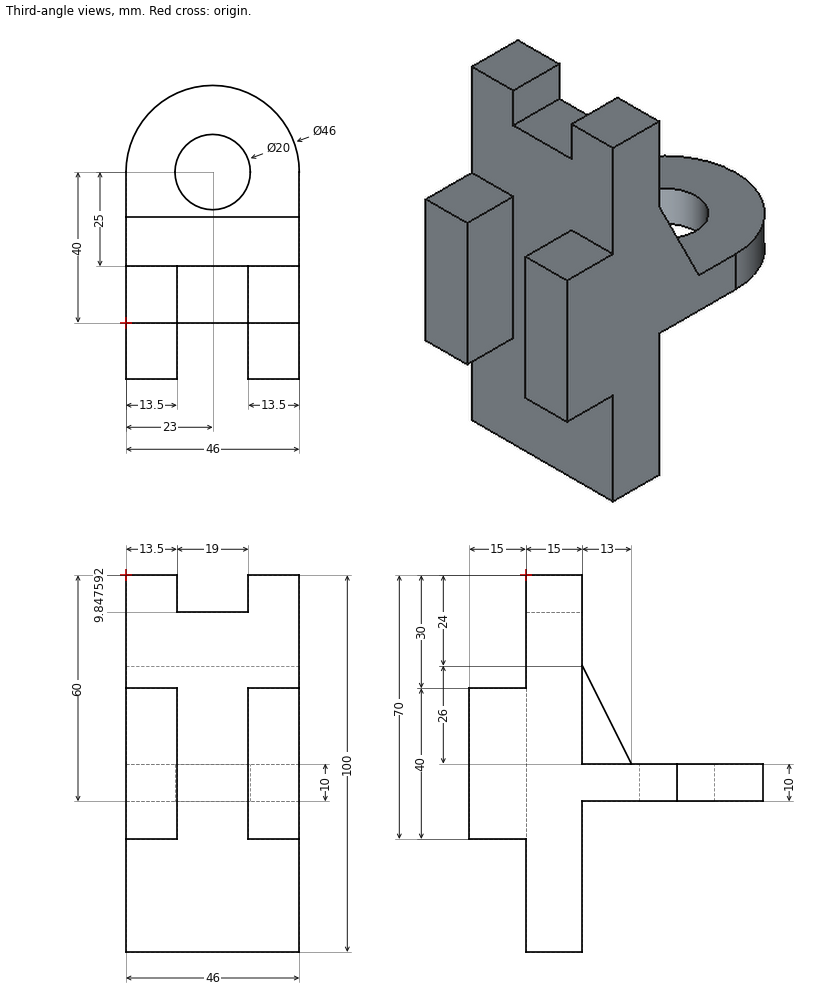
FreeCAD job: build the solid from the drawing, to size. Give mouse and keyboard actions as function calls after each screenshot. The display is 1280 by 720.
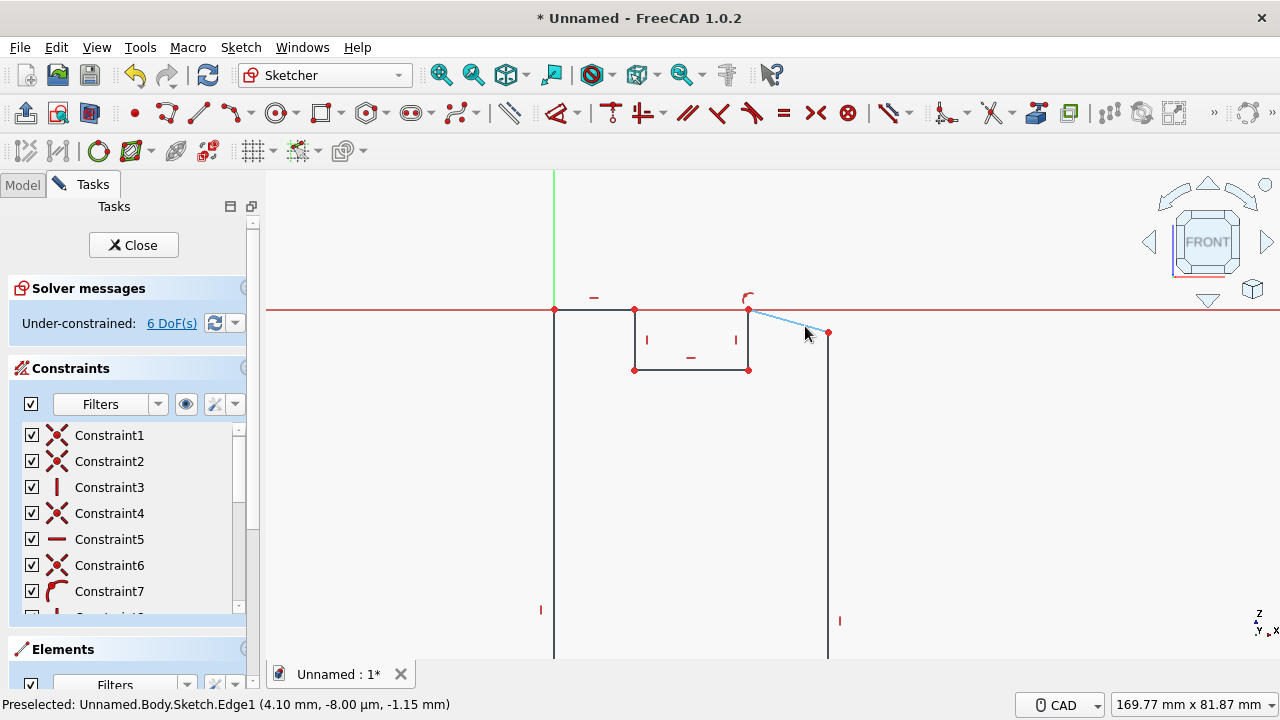
click(804, 325)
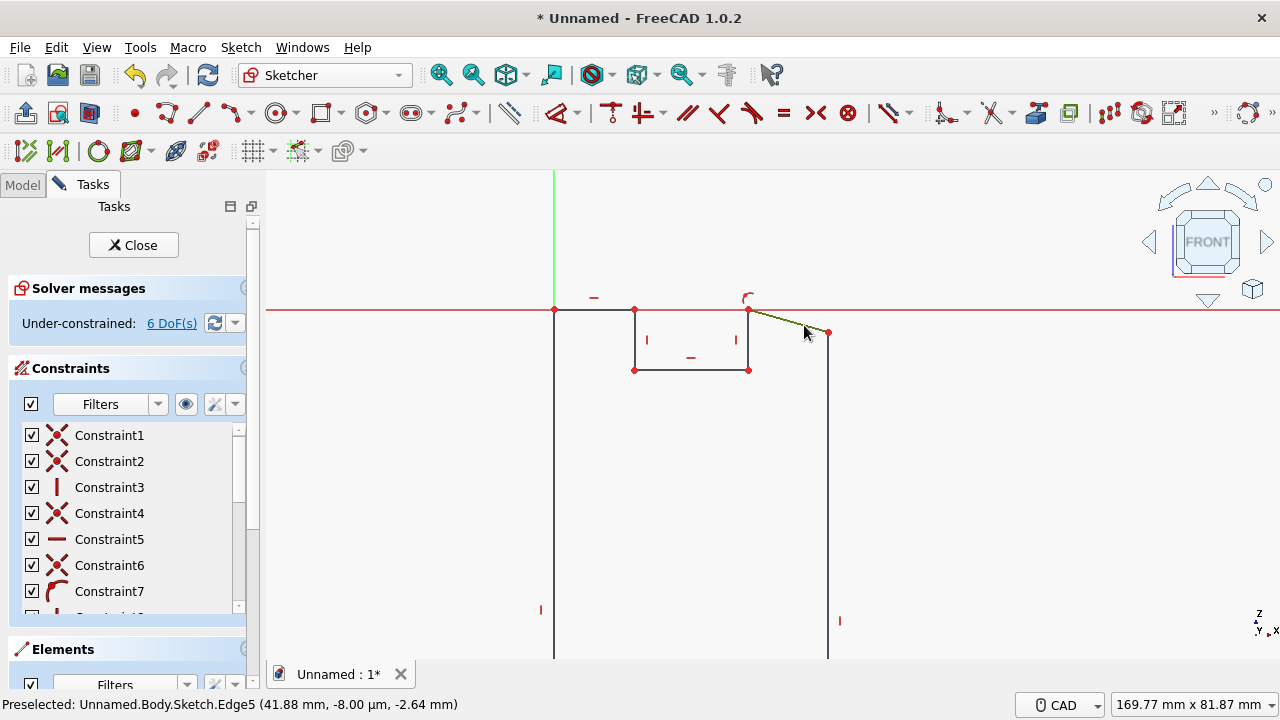
key(h)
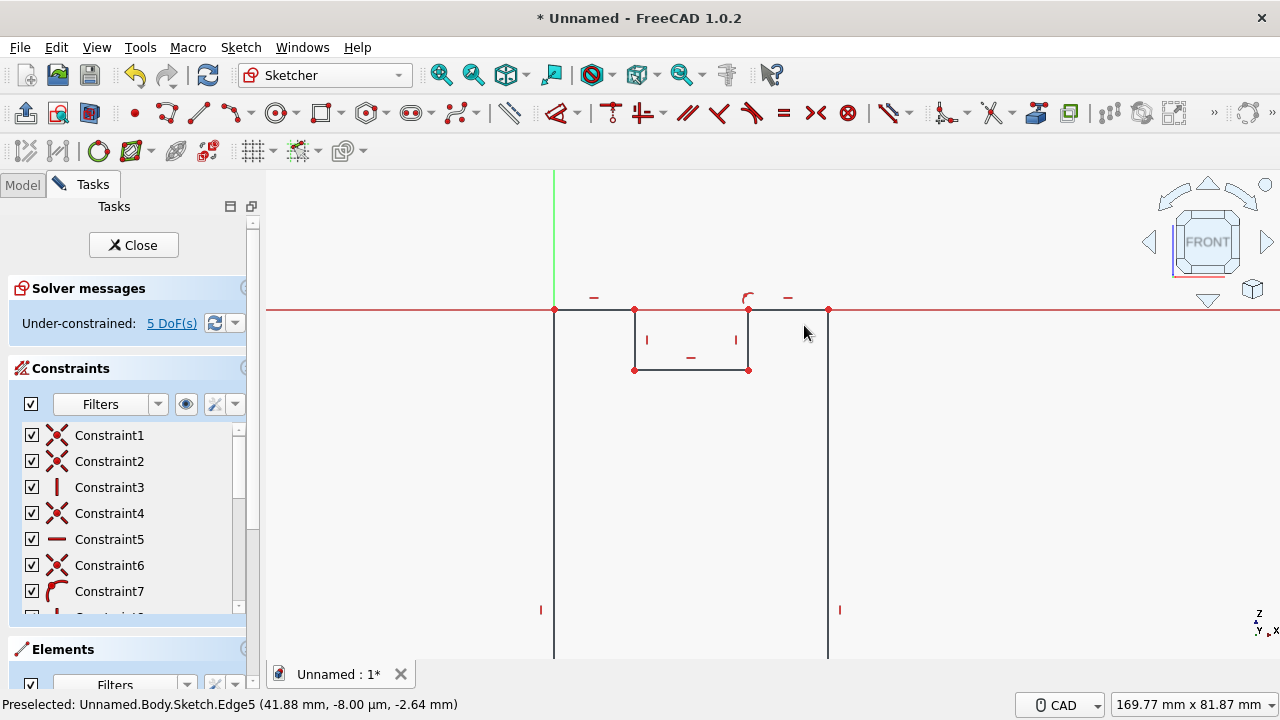
key(d)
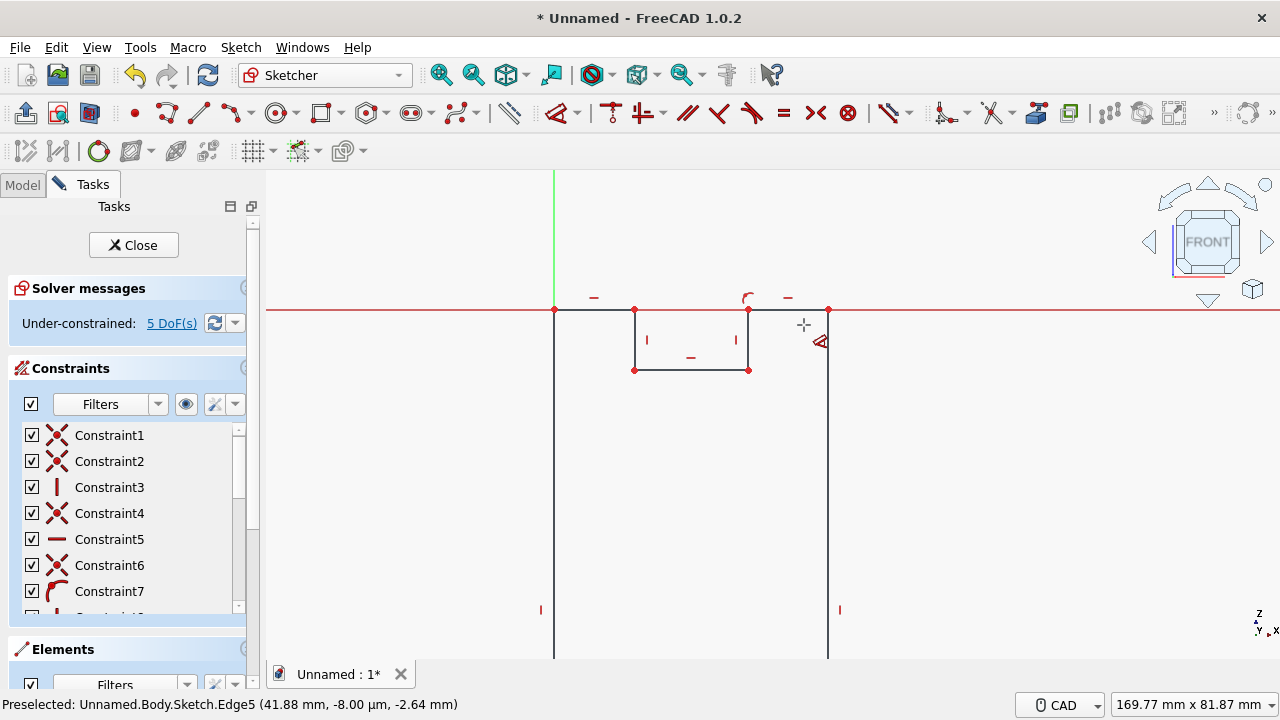
click(669, 370)
click(692, 336)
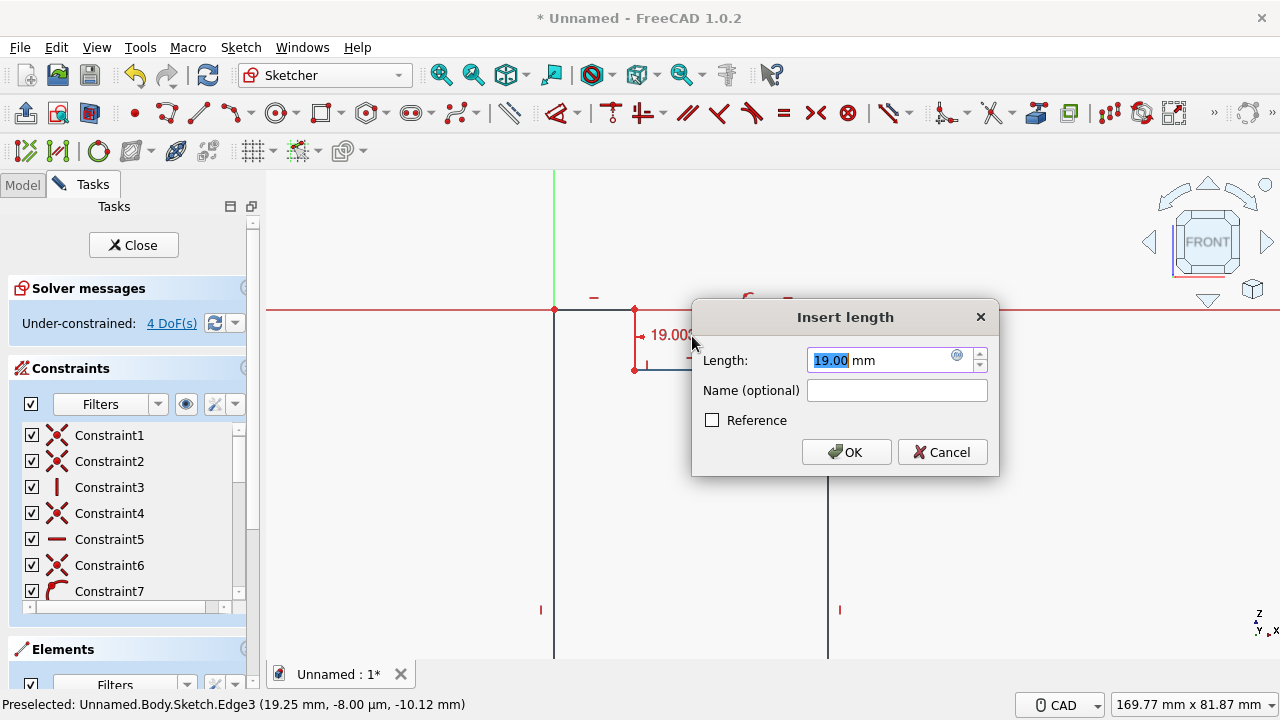
text(19)
key(Return)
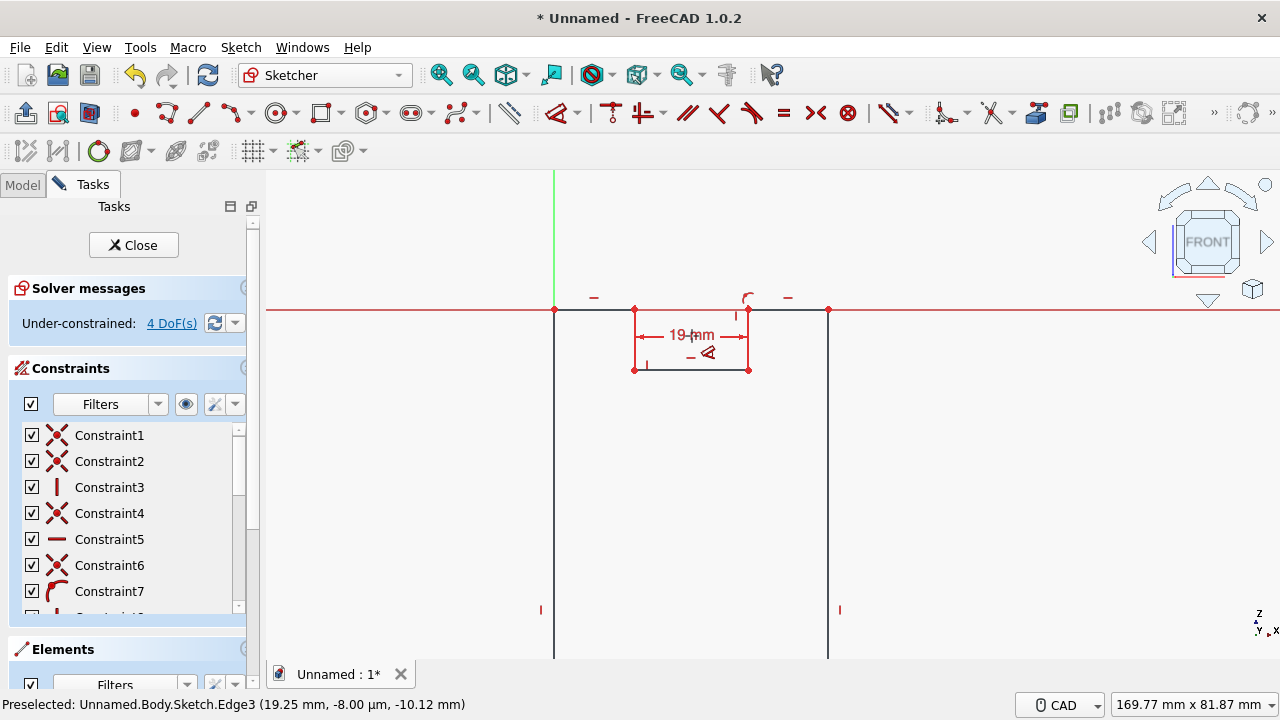
scroll(720, 198, down, 3)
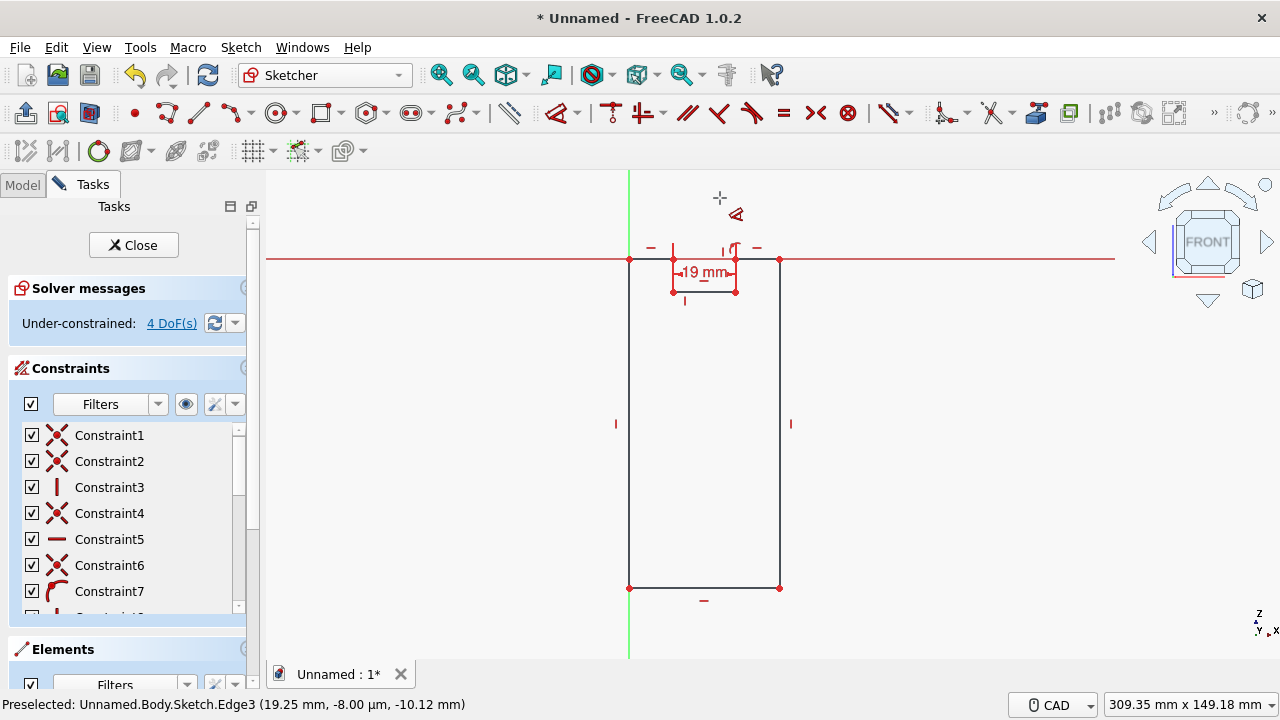
click(735, 588)
click(704, 622)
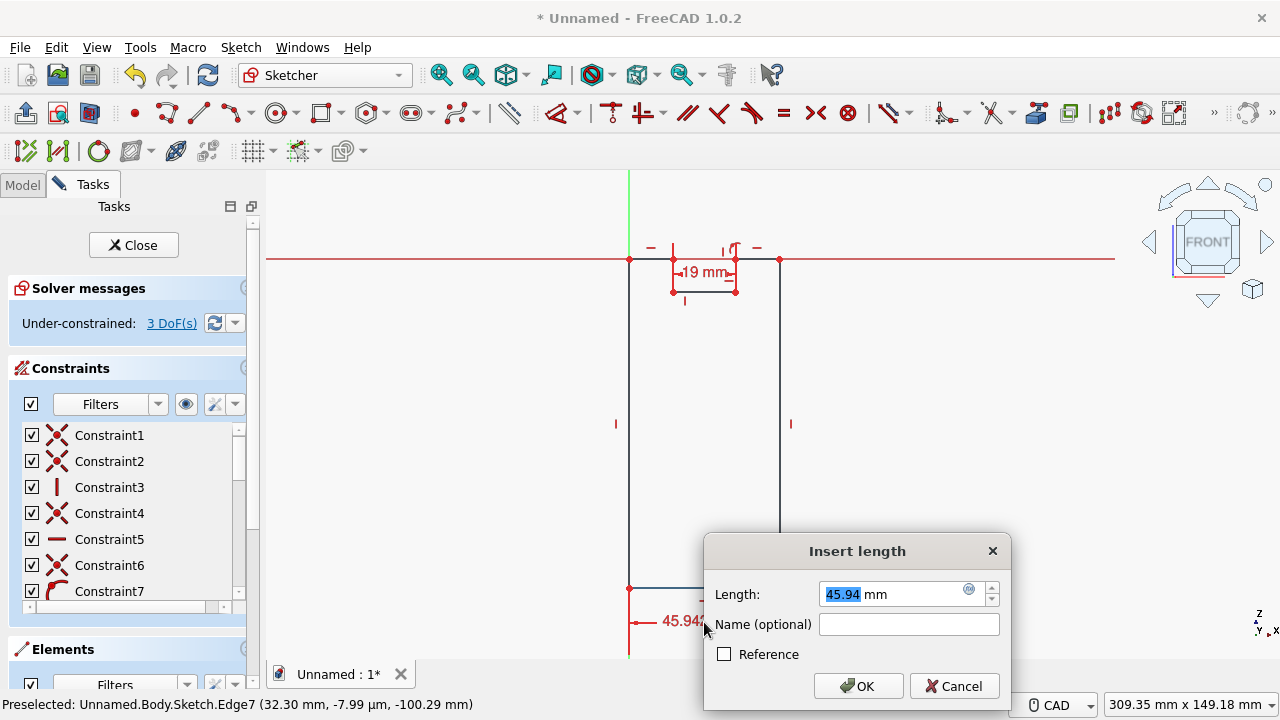
text(46)
key(Return)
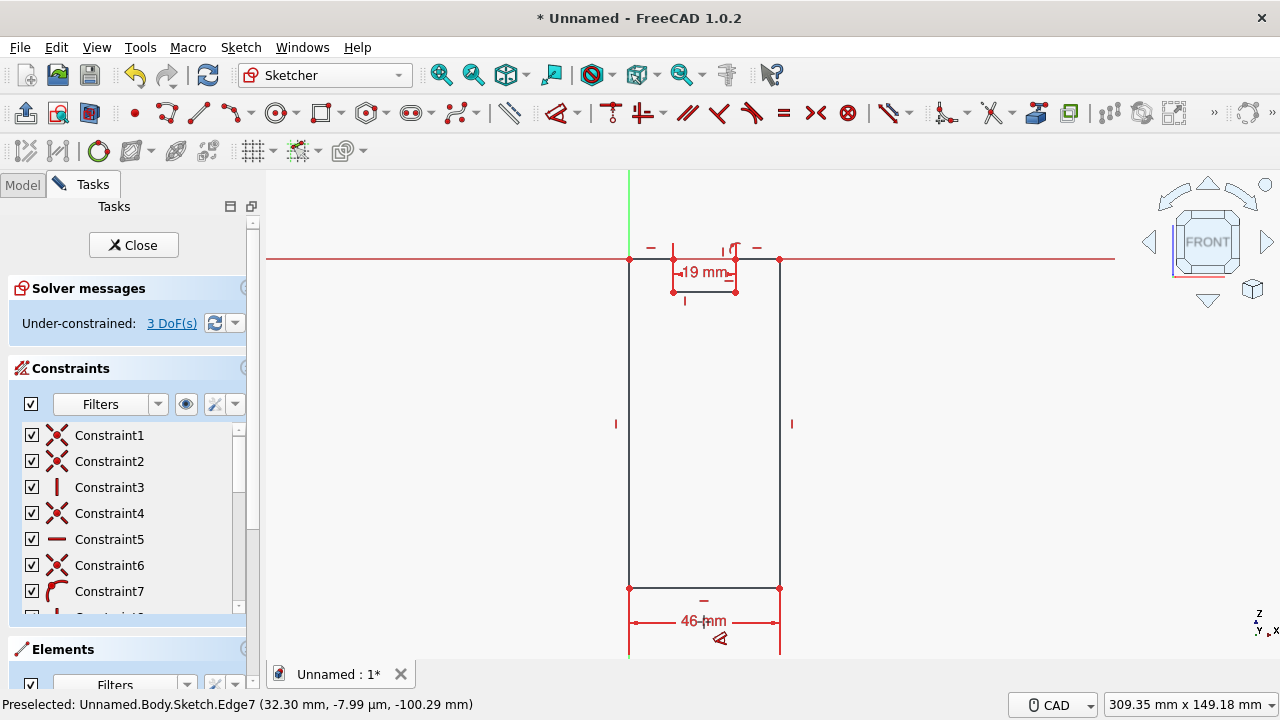
click(780, 358)
click(814, 424)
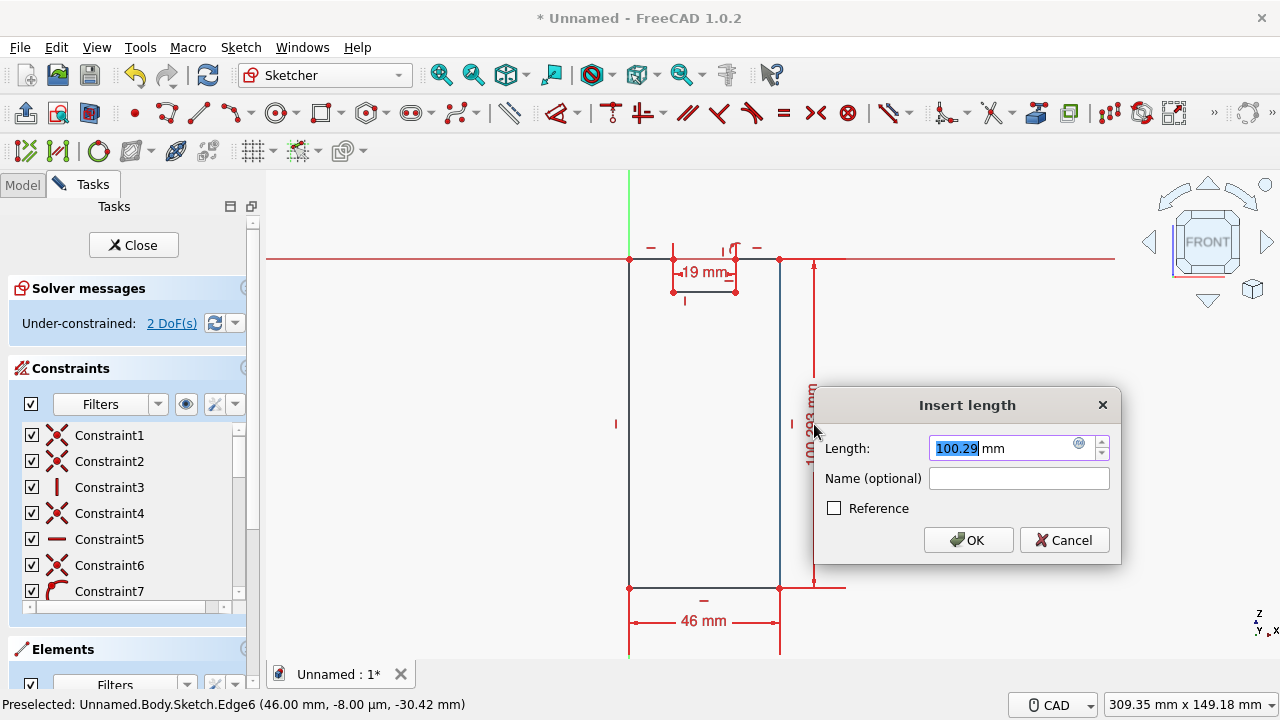
text(100)
key(Return)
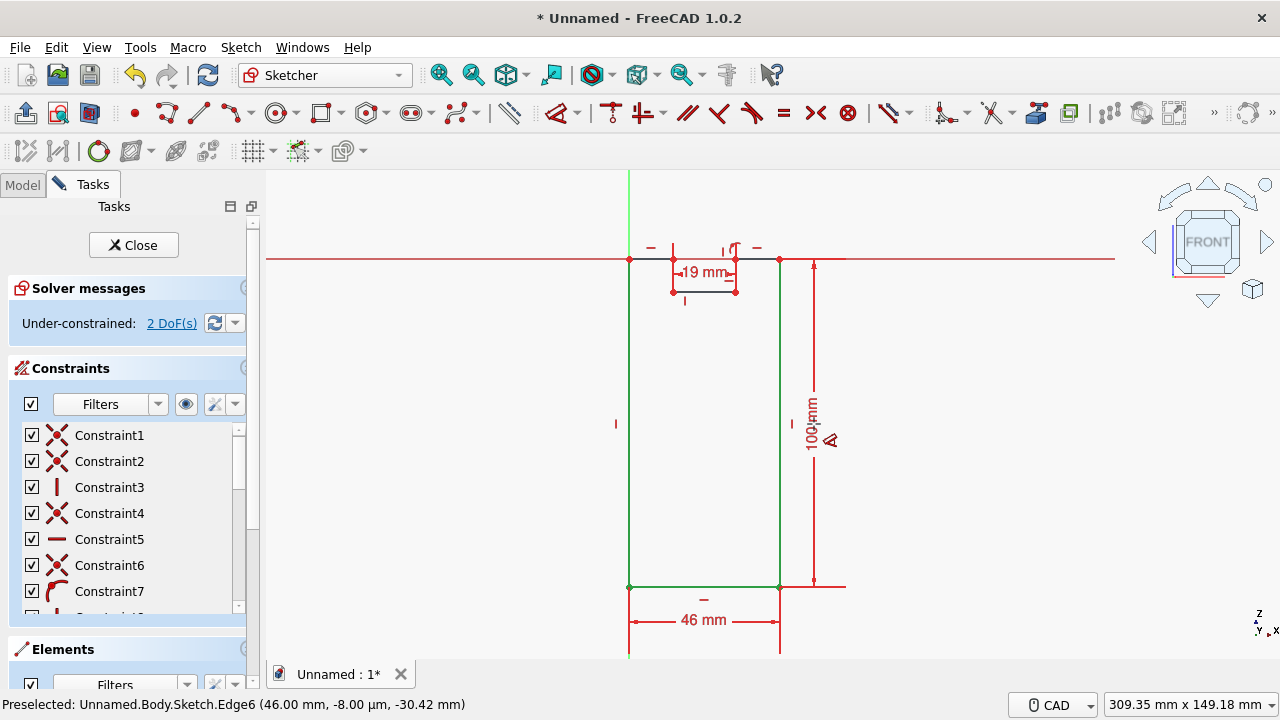
click(642, 259)
click(651, 225)